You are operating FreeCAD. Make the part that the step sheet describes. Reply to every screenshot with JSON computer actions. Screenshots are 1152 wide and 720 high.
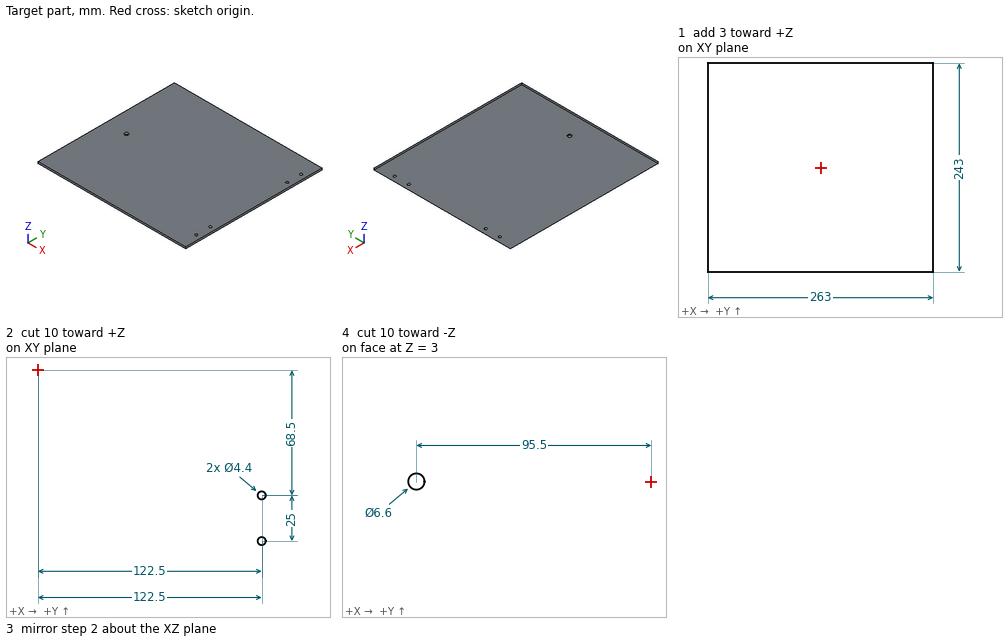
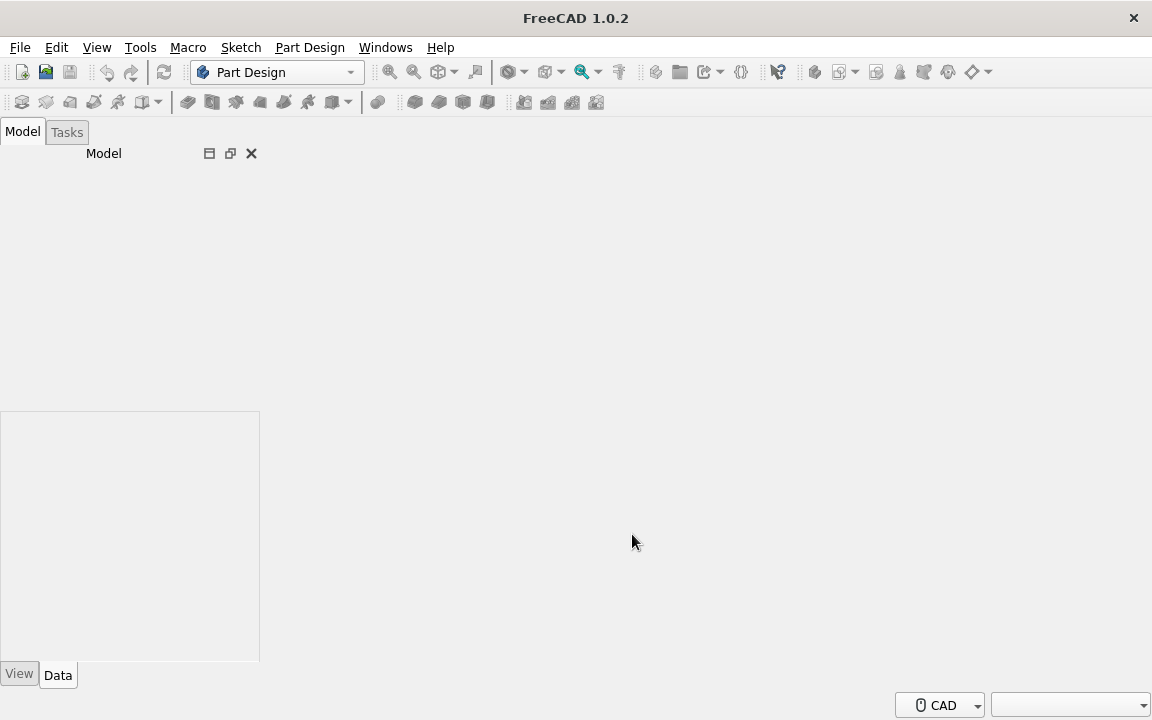
{"action": "key", "text": "ctrl+n"}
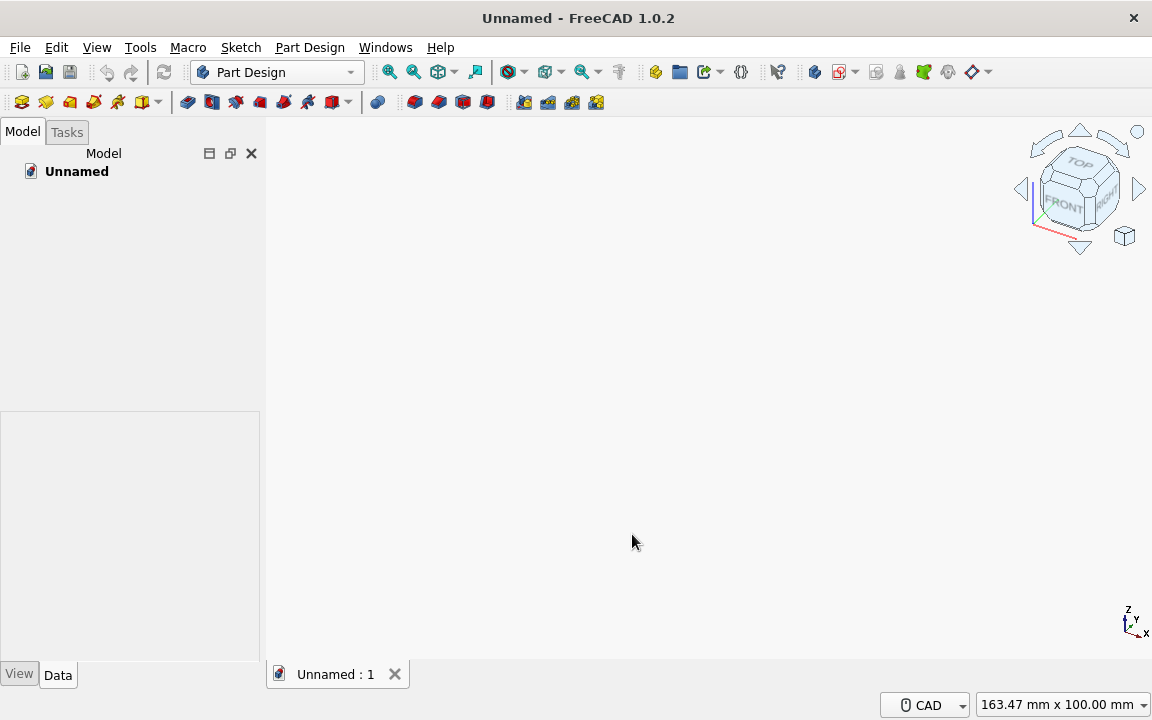
{"action": "left_click", "coordinate": [840, 72]}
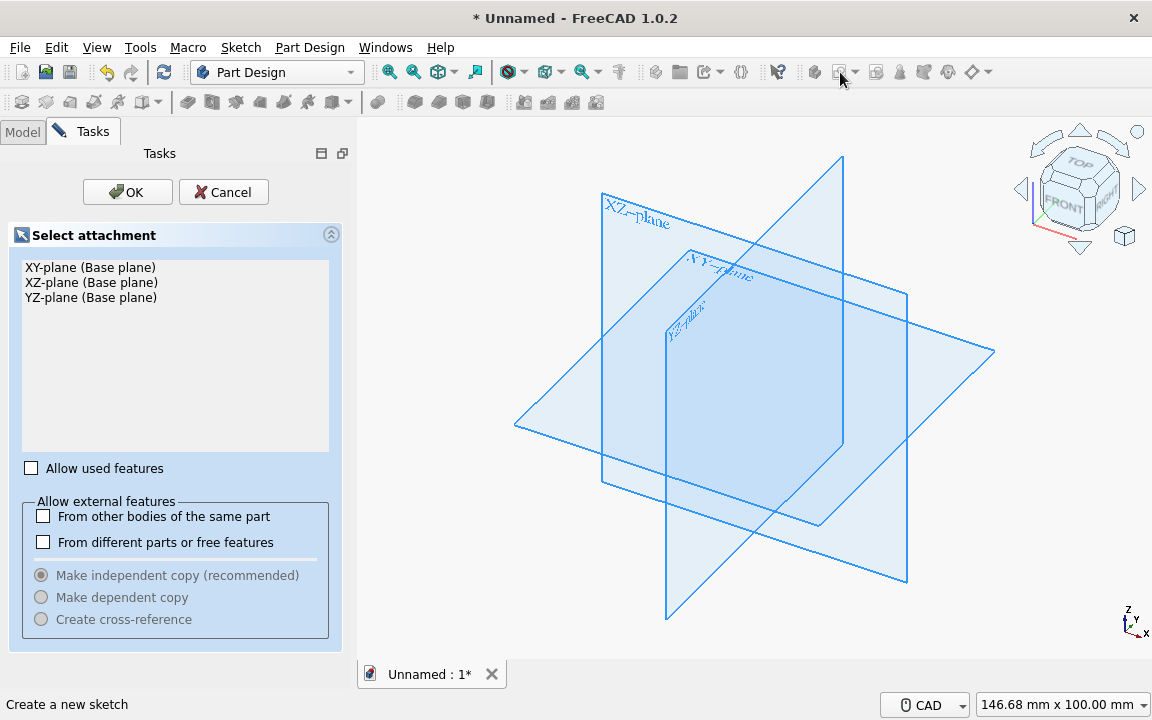
{"action": "left_click", "coordinate": [82, 268]}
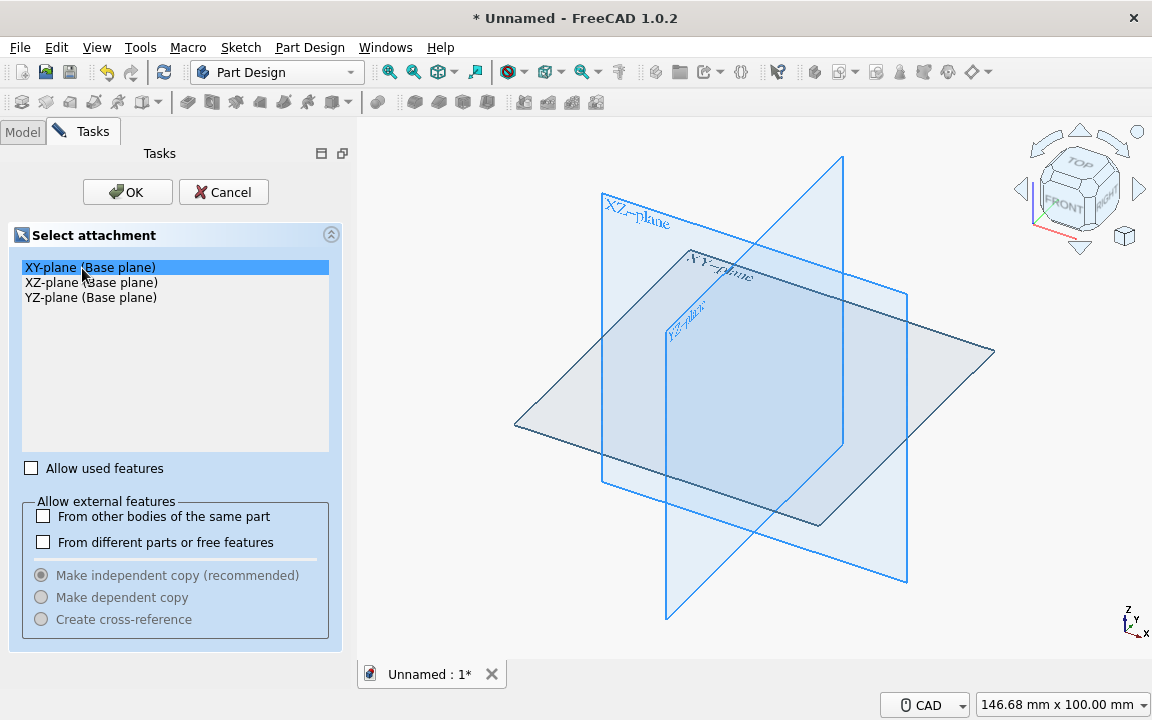
{"action": "left_click", "coordinate": [128, 192]}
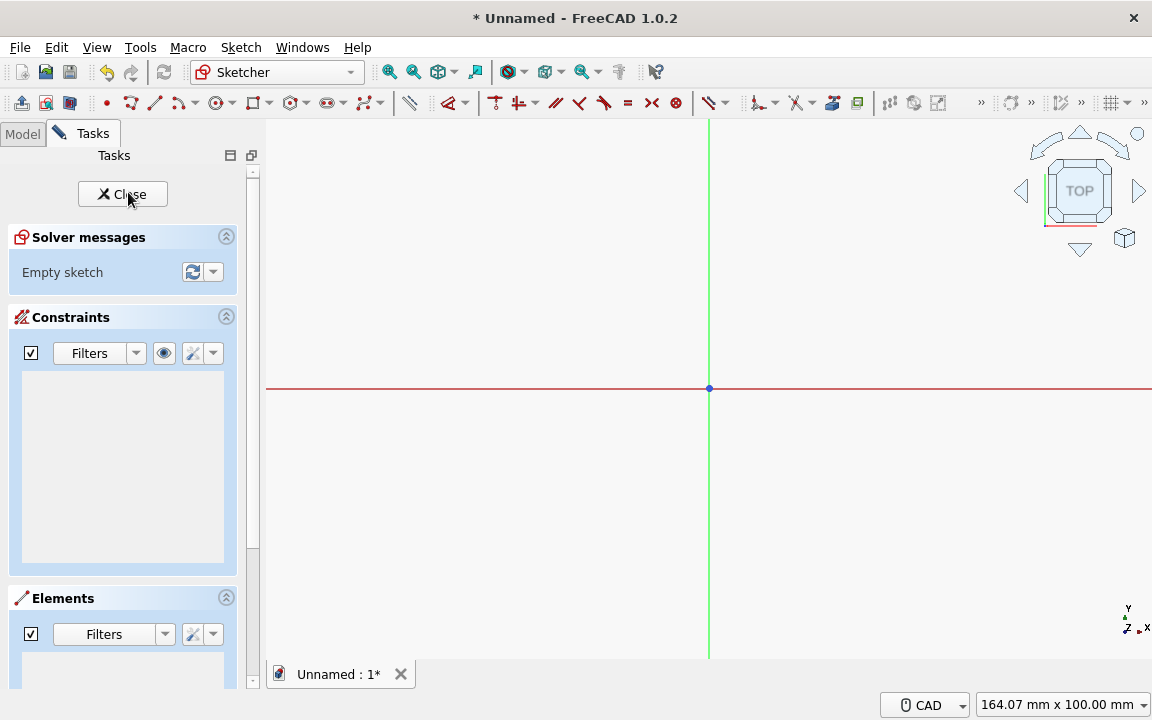
{"action": "scroll", "coordinate": [618, 389], "scroll_direction": "down", "scroll_amount": 7}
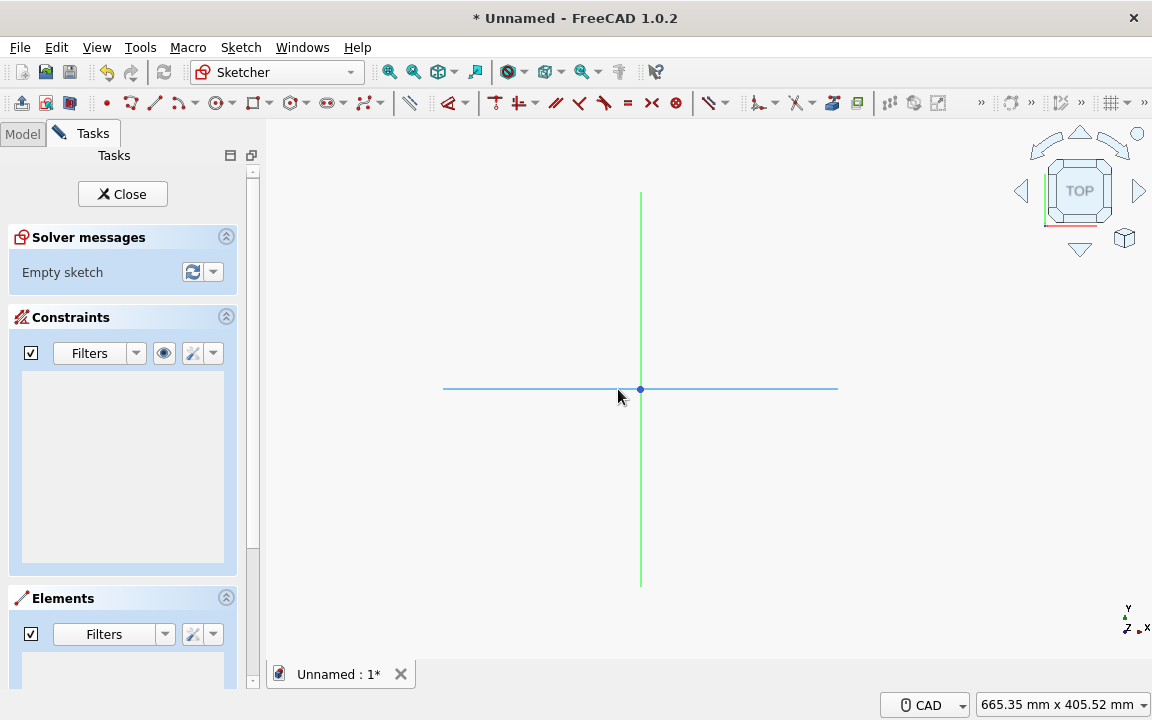
{"action": "key", "text": "g v"}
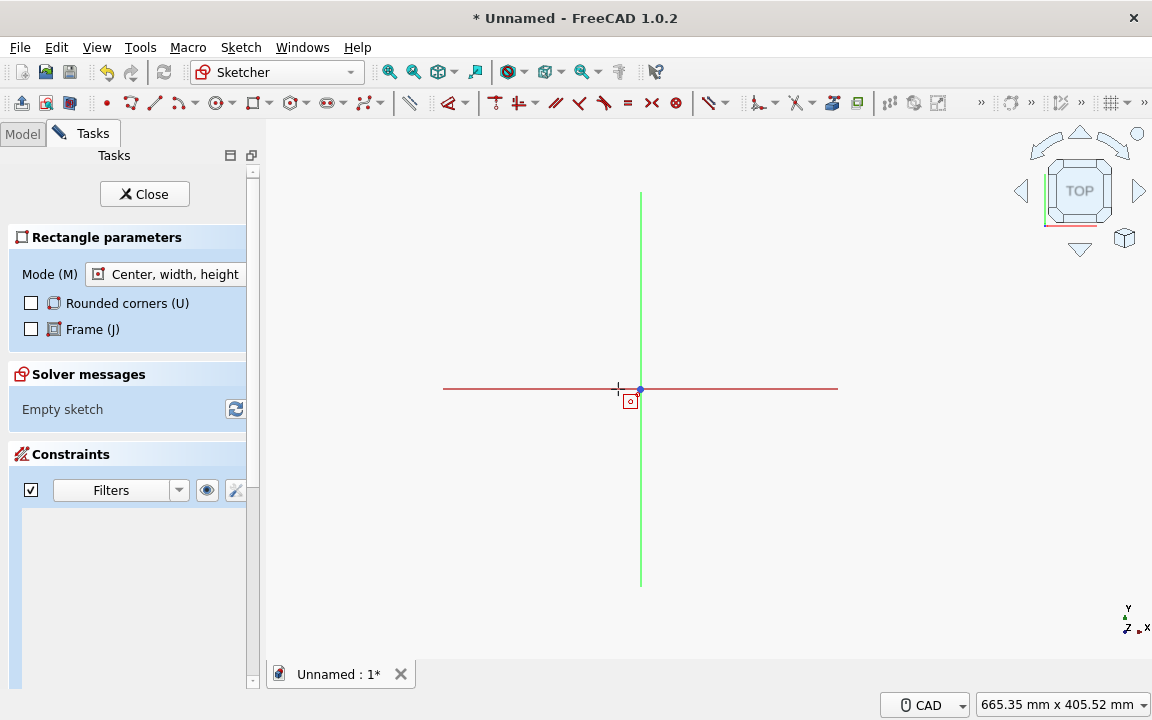
{"action": "left_click", "coordinate": [641, 389]}
{"action": "left_click", "coordinate": [816, 228]}
{"action": "key", "text": "Escape"}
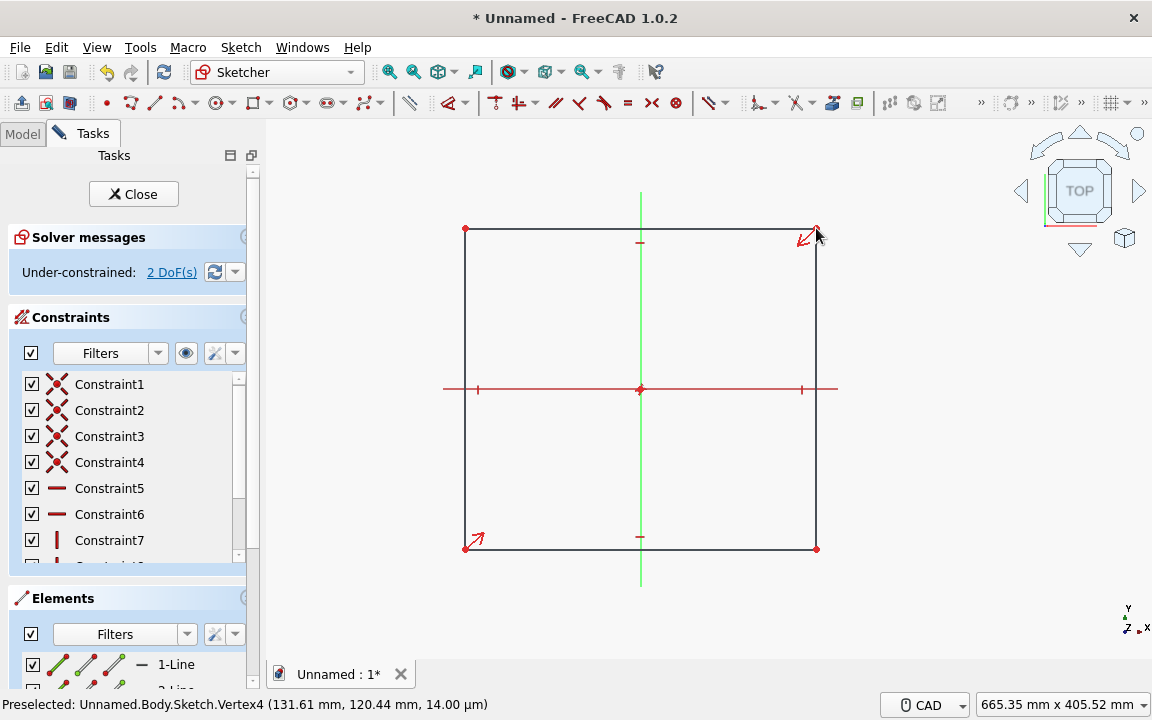
{"action": "left_click", "coordinate": [571, 550]}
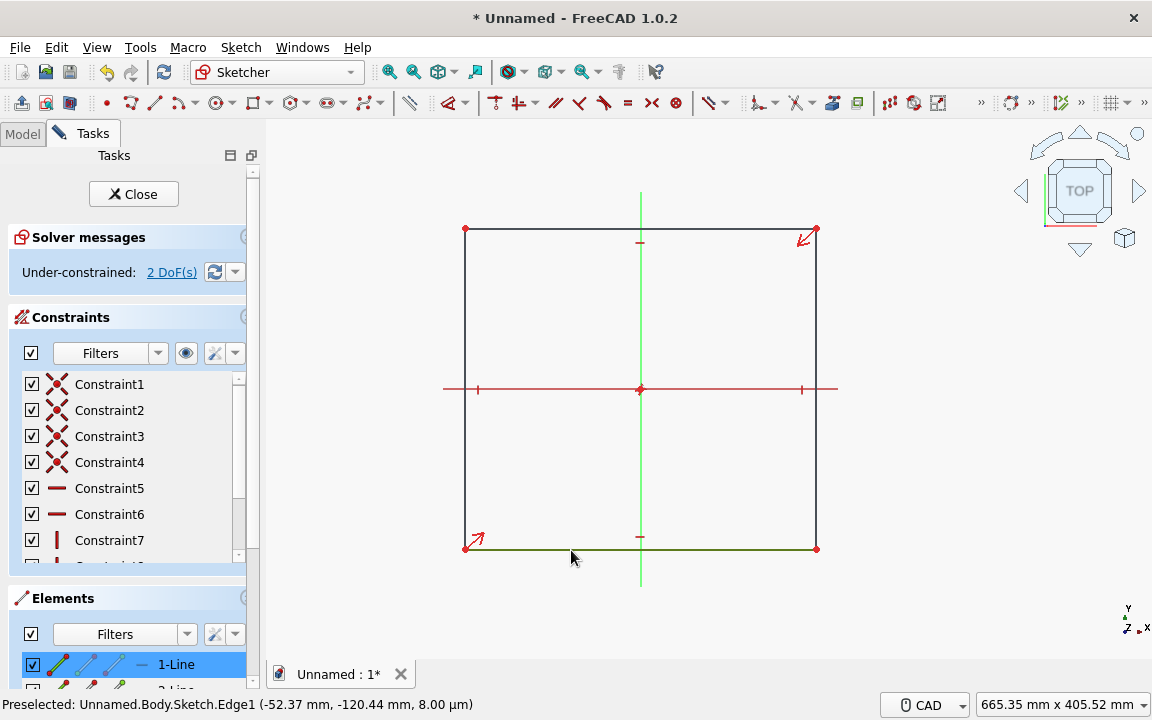
{"action": "key", "text": "l"}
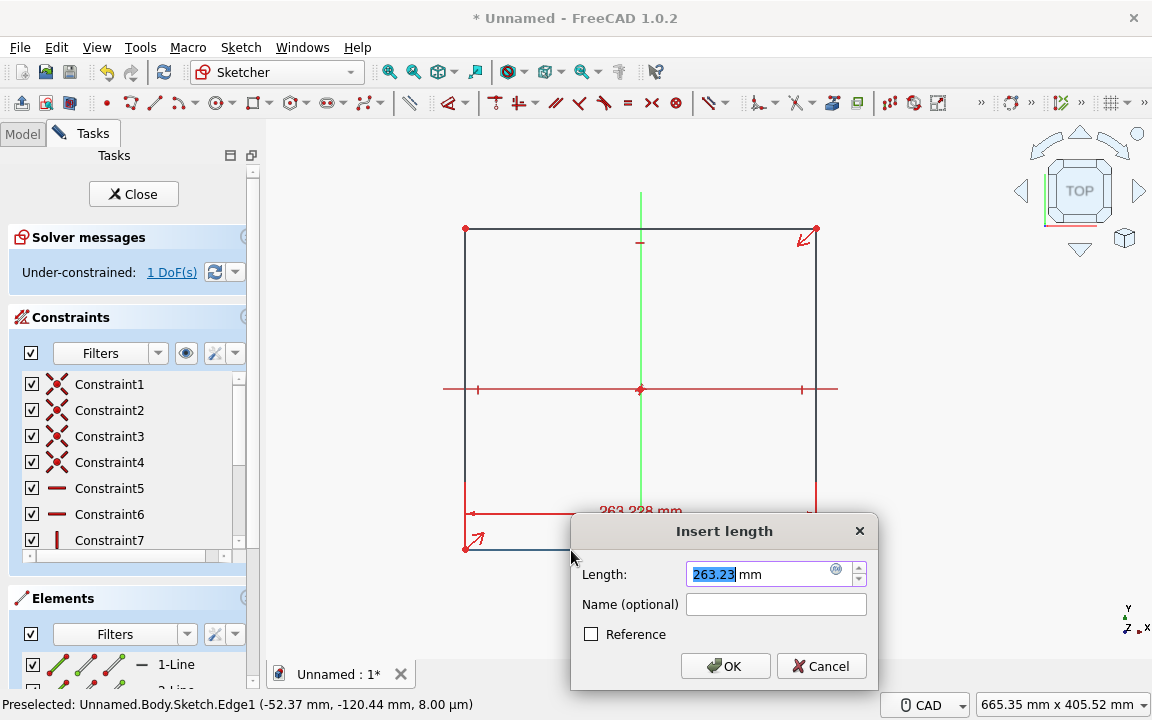
{"action": "type", "text": "263"}
{"action": "key", "text": "Return"}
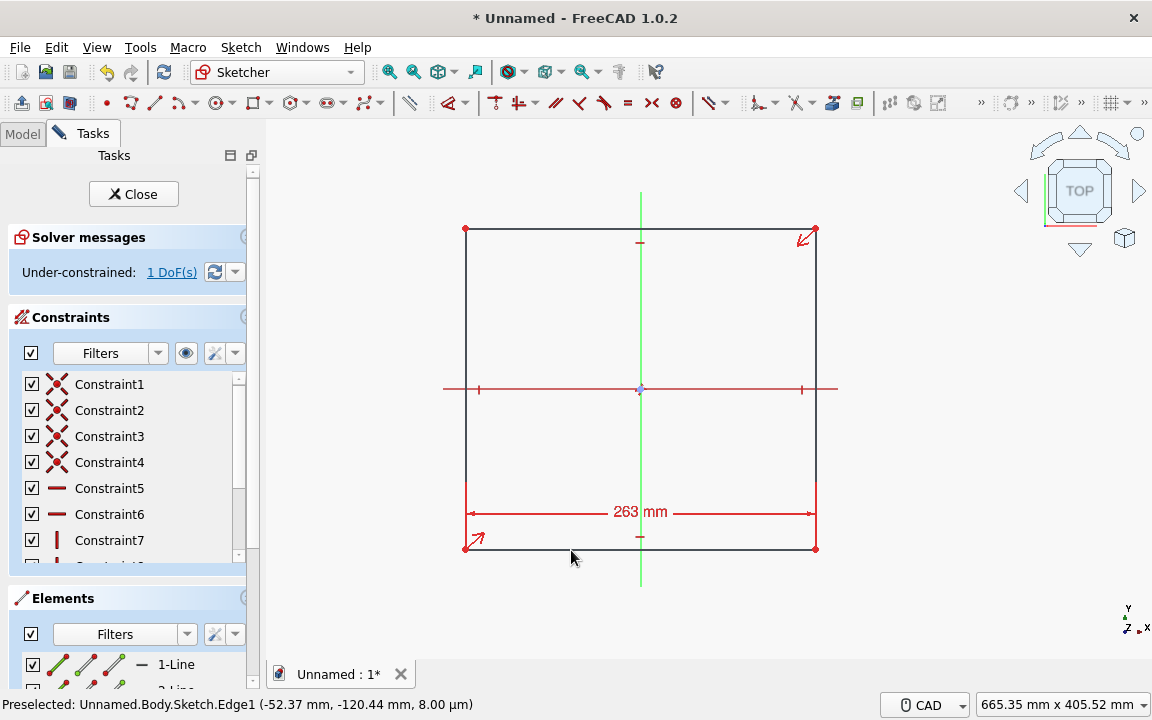
{"action": "left_click", "coordinate": [816, 454]}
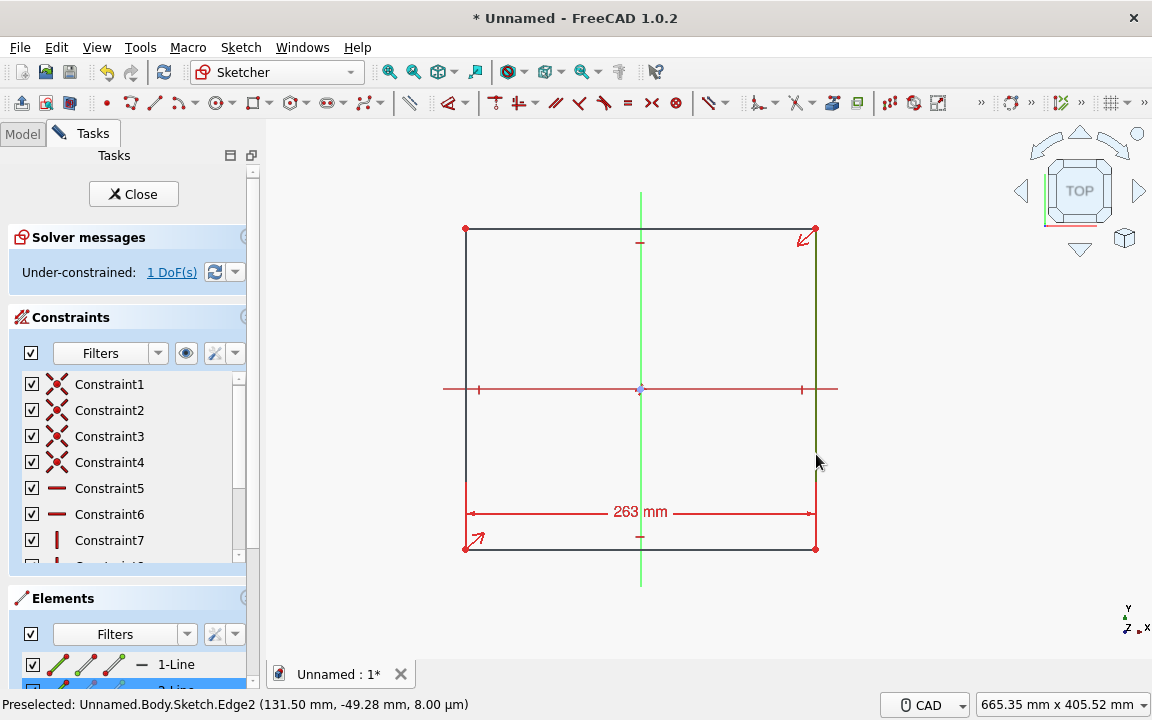
{"action": "key", "text": "i"}